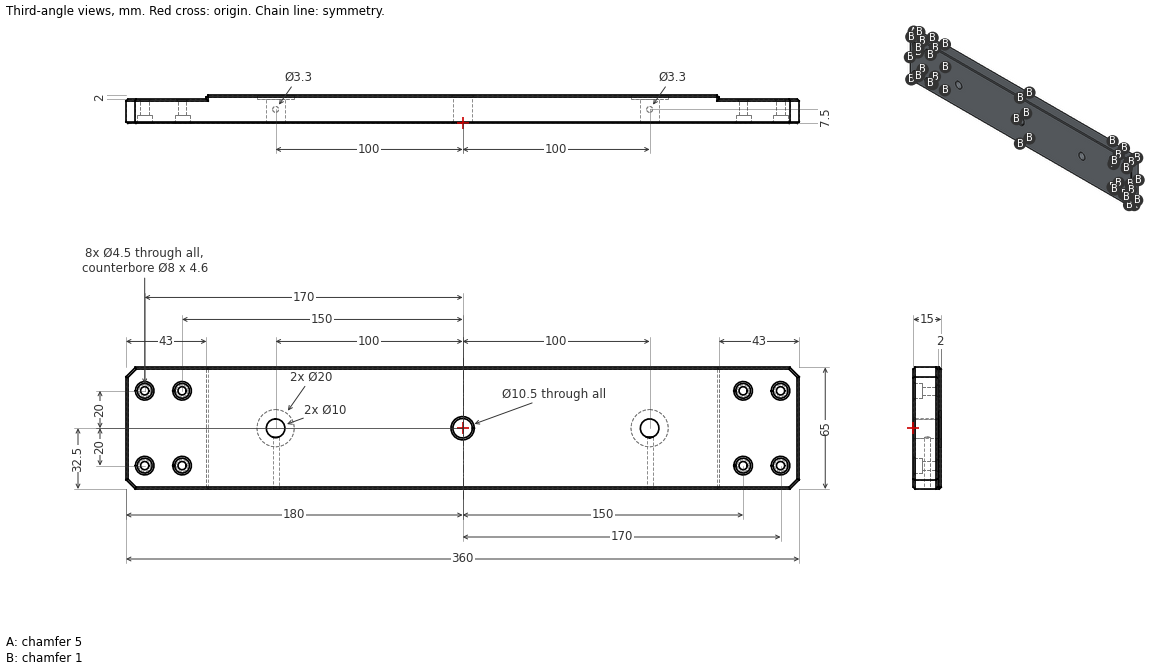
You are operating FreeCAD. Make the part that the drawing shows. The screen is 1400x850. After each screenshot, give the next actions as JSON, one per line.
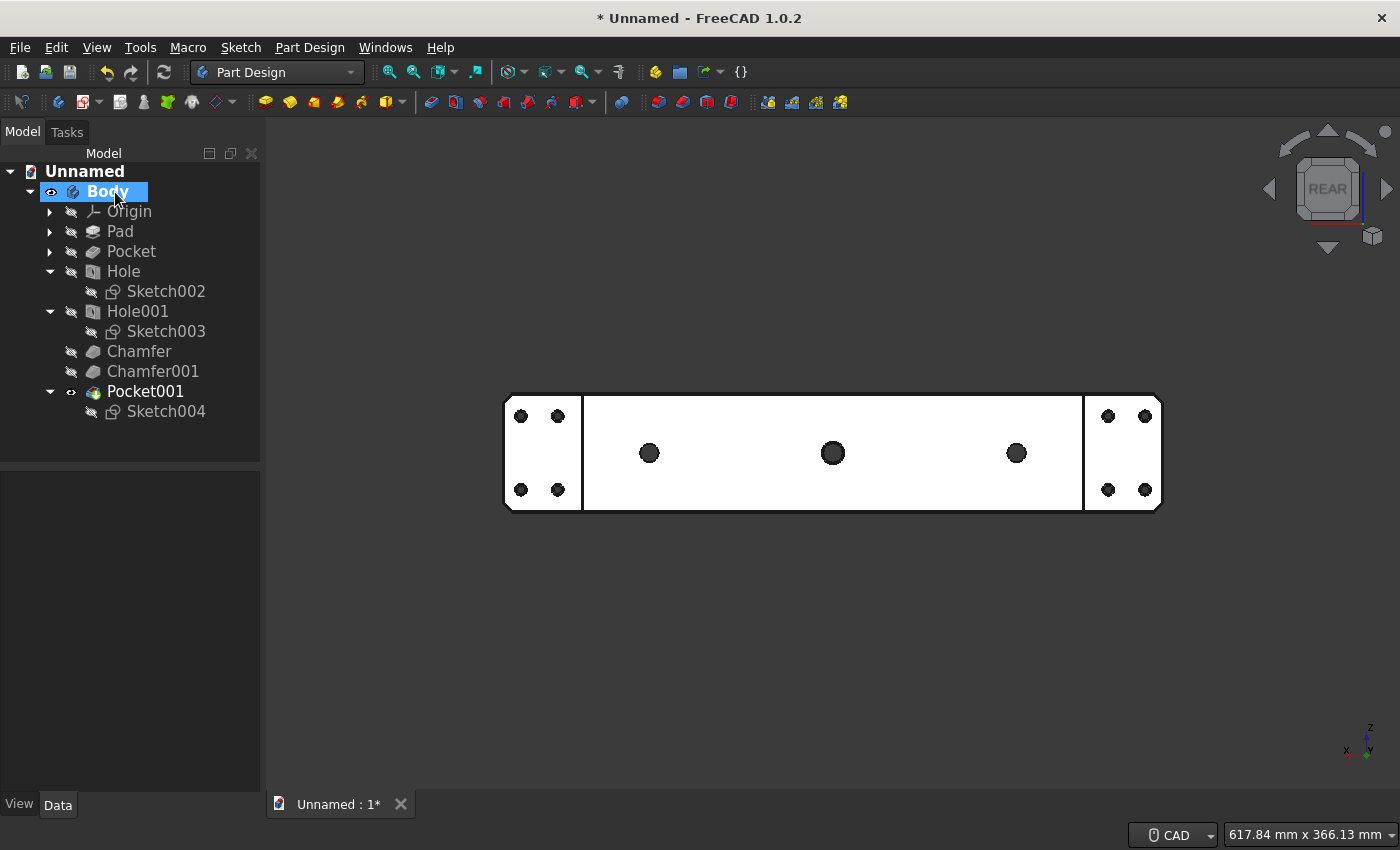
{"action": "key", "text": "5"}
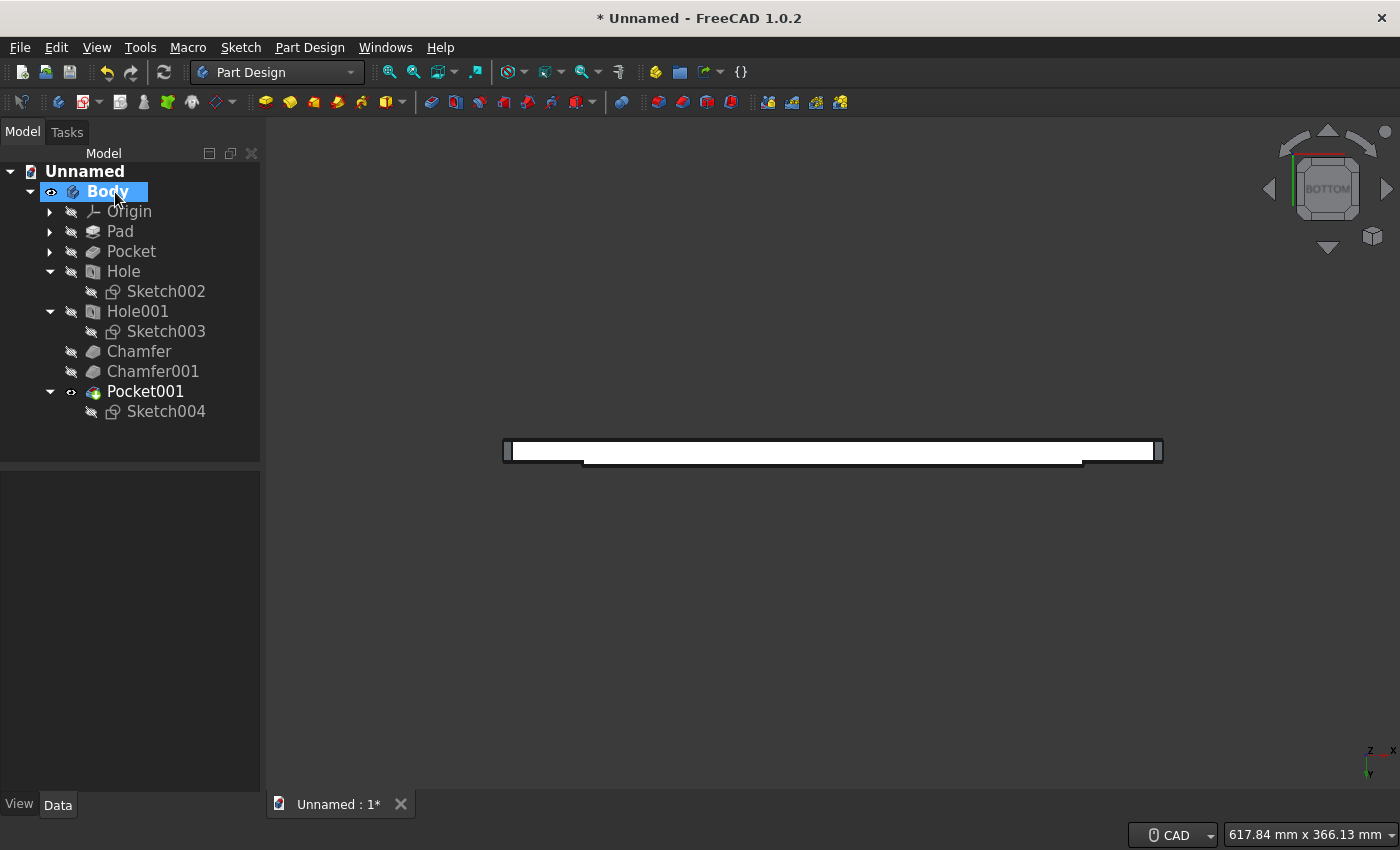
{"action": "left_click", "coordinate": [1017, 452]}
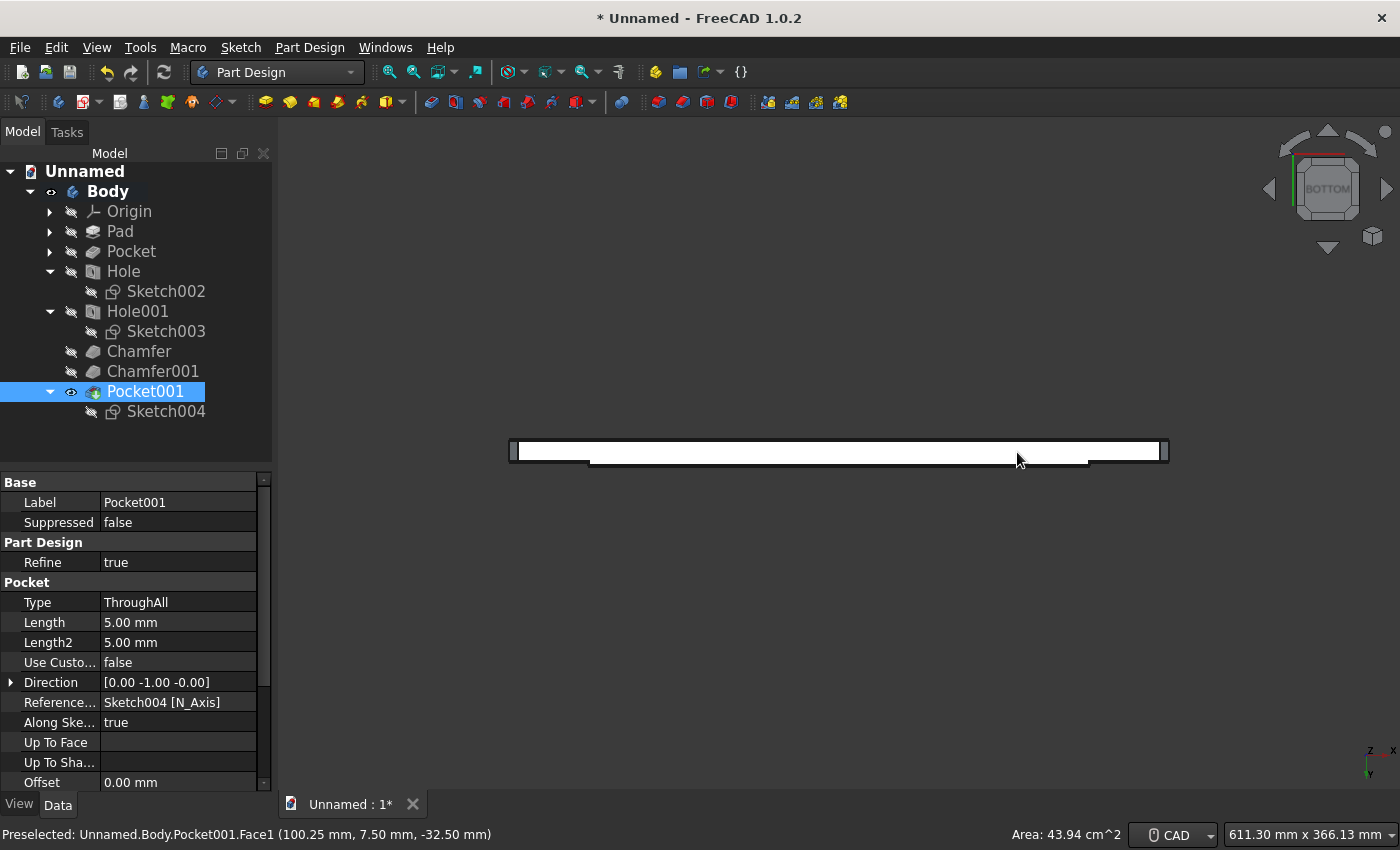
{"action": "left_click", "coordinate": [84, 102]}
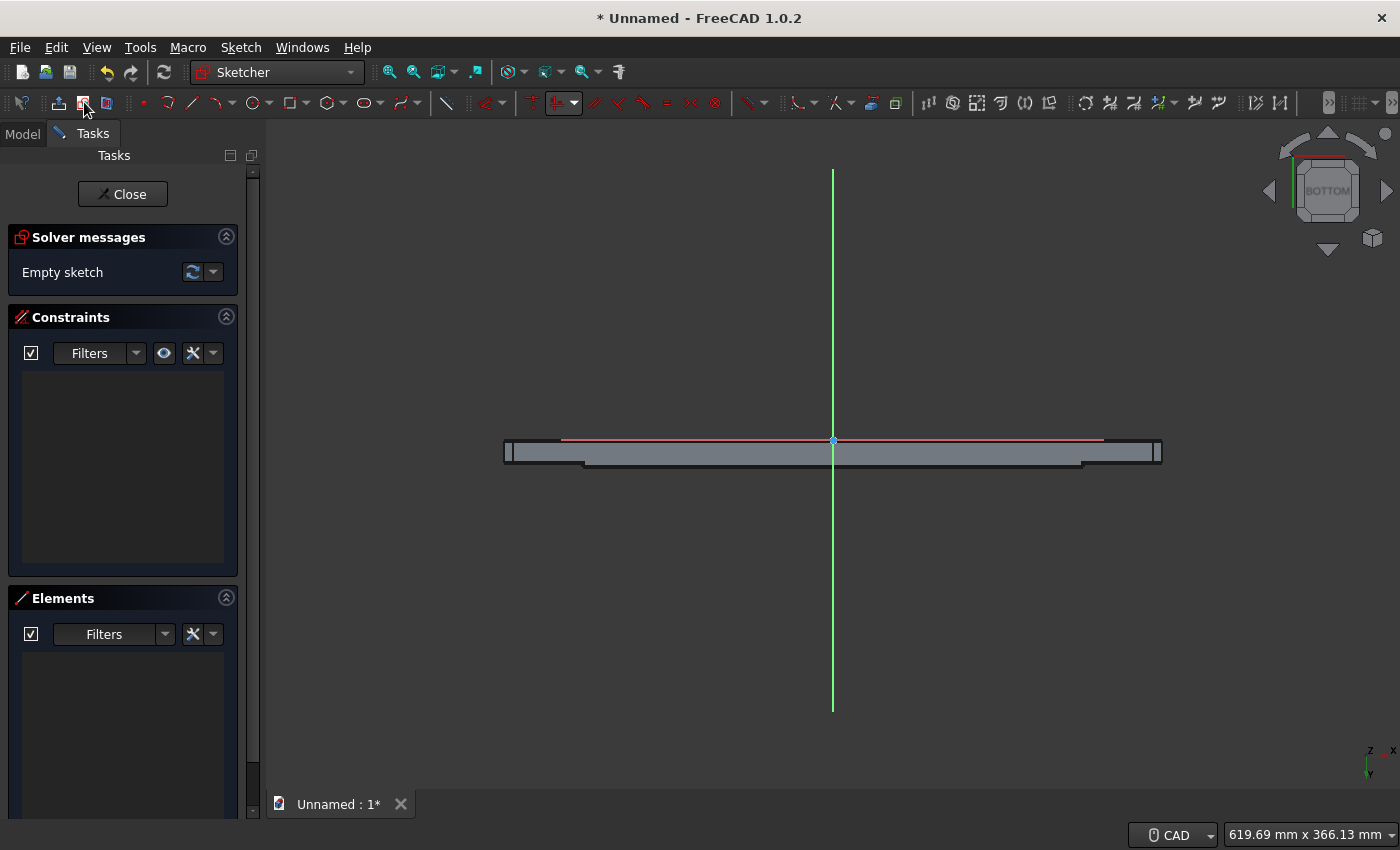
{"action": "scroll", "coordinate": [1029, 454], "scroll_direction": "up", "scroll_amount": 15}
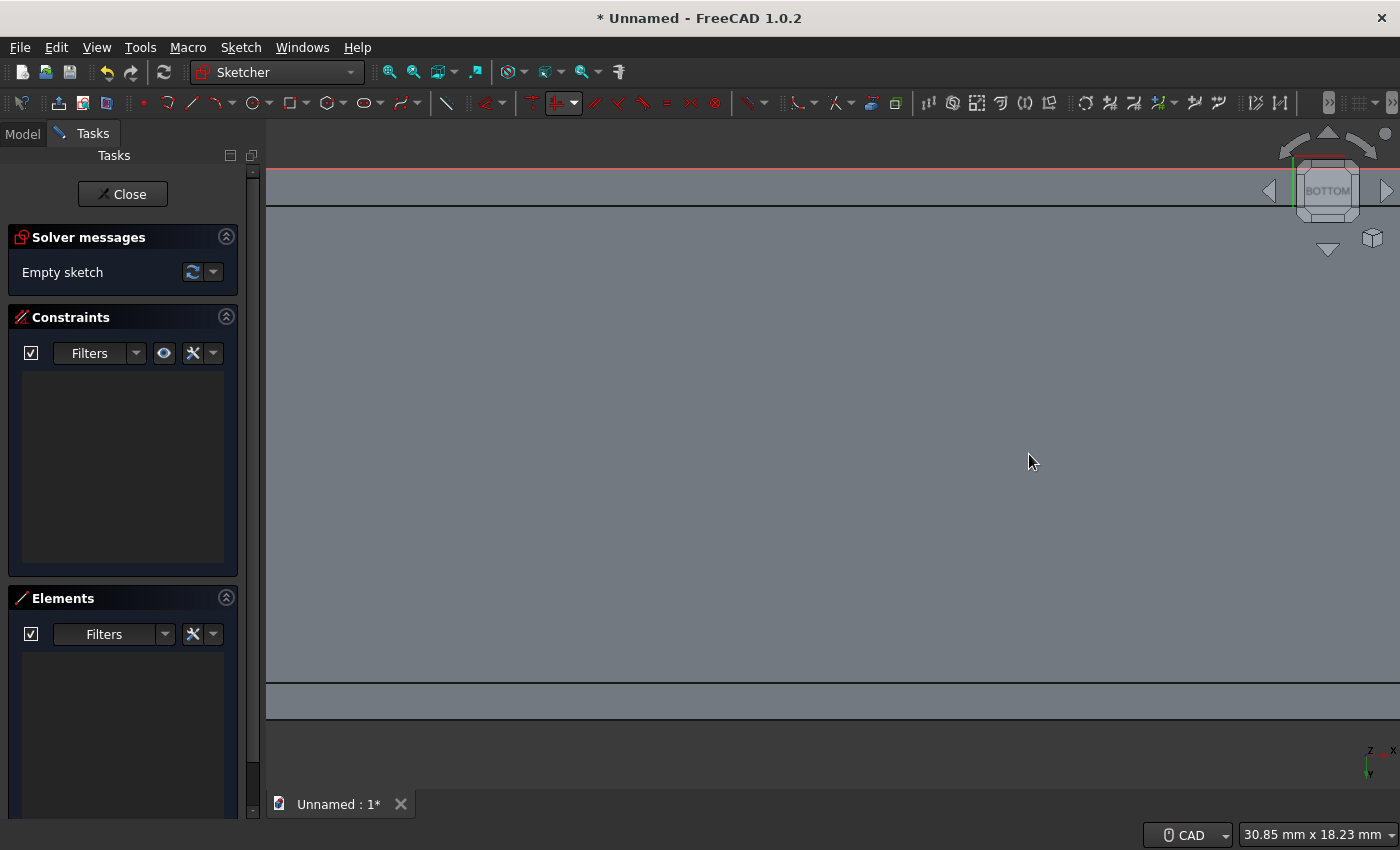
{"action": "scroll", "coordinate": [751, 440], "scroll_direction": "up", "scroll_amount": 6}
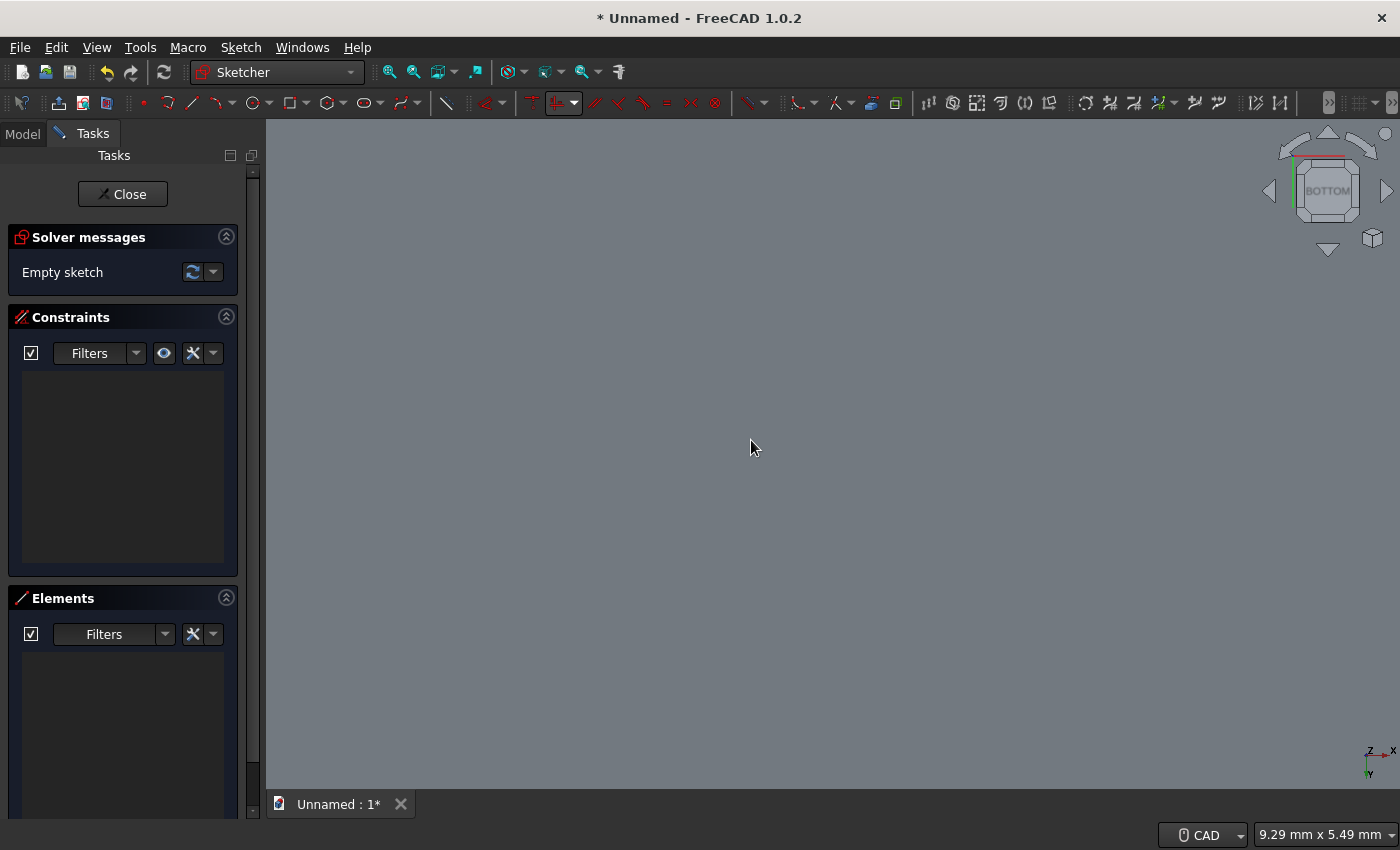
{"action": "left_click", "coordinate": [254, 104]}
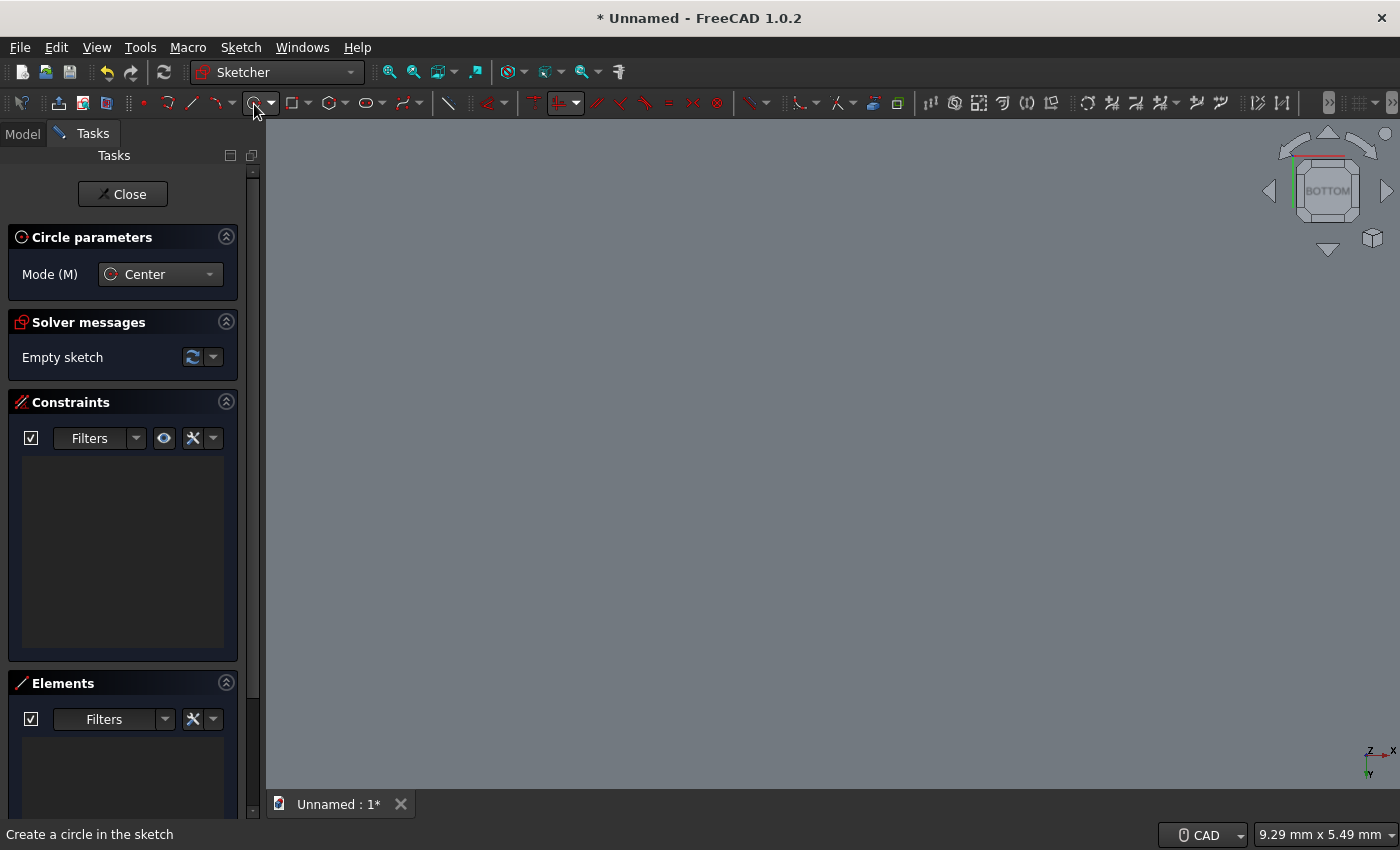
{"action": "left_click", "coordinate": [763, 454]}
{"action": "mouse_move", "coordinate": [906, 311]}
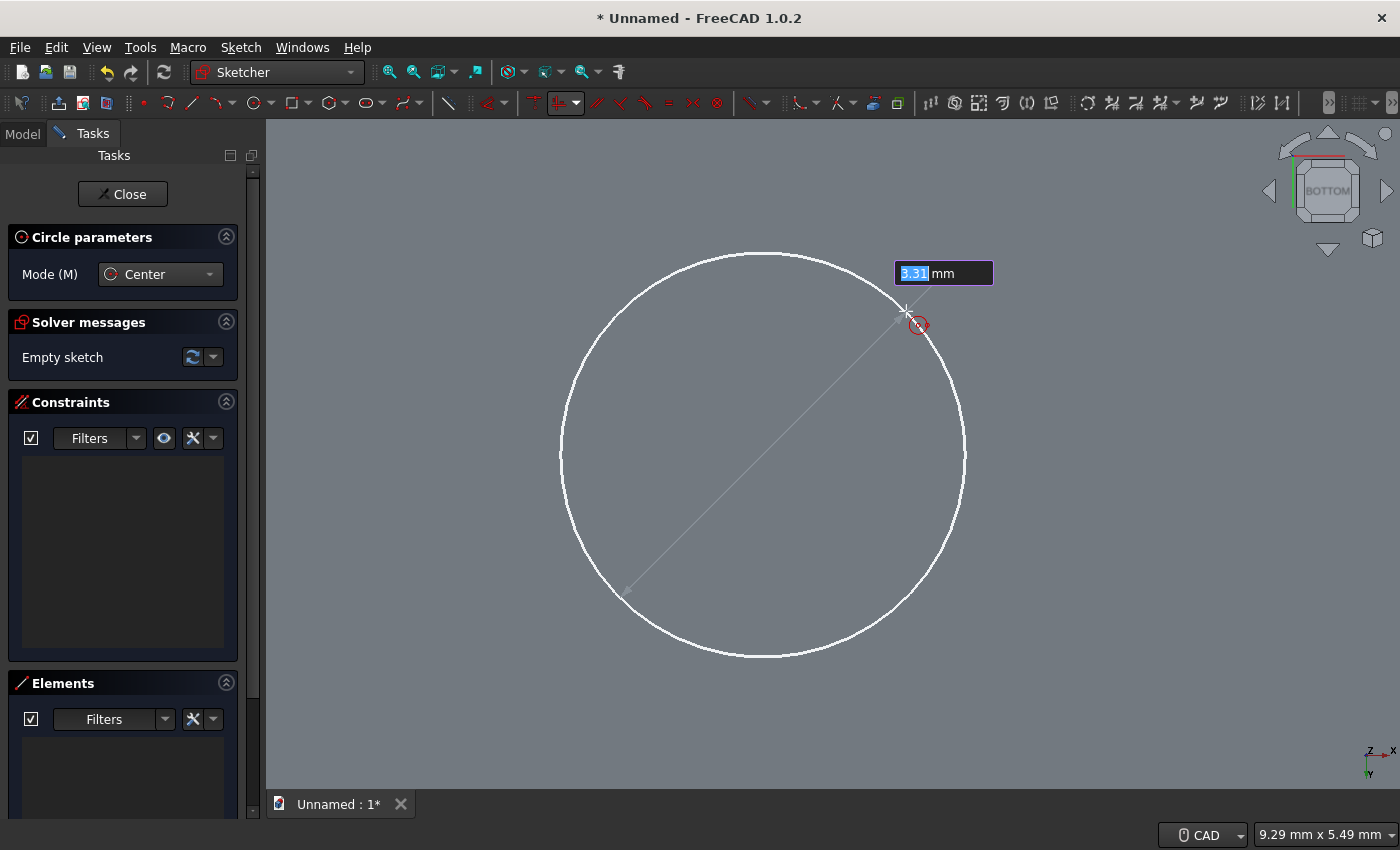
{"action": "type", "text": "3.3"}
{"action": "key", "text": "Return"}
{"action": "key", "text": "Escape"}